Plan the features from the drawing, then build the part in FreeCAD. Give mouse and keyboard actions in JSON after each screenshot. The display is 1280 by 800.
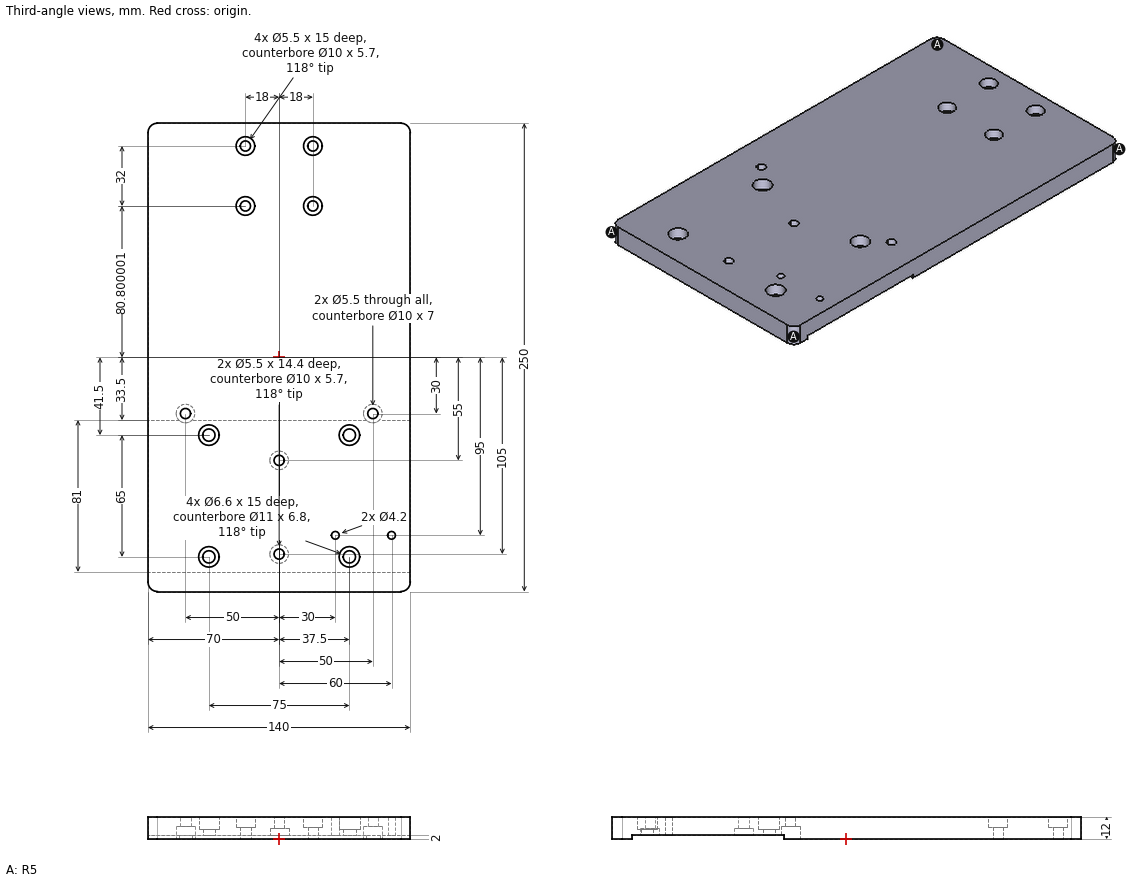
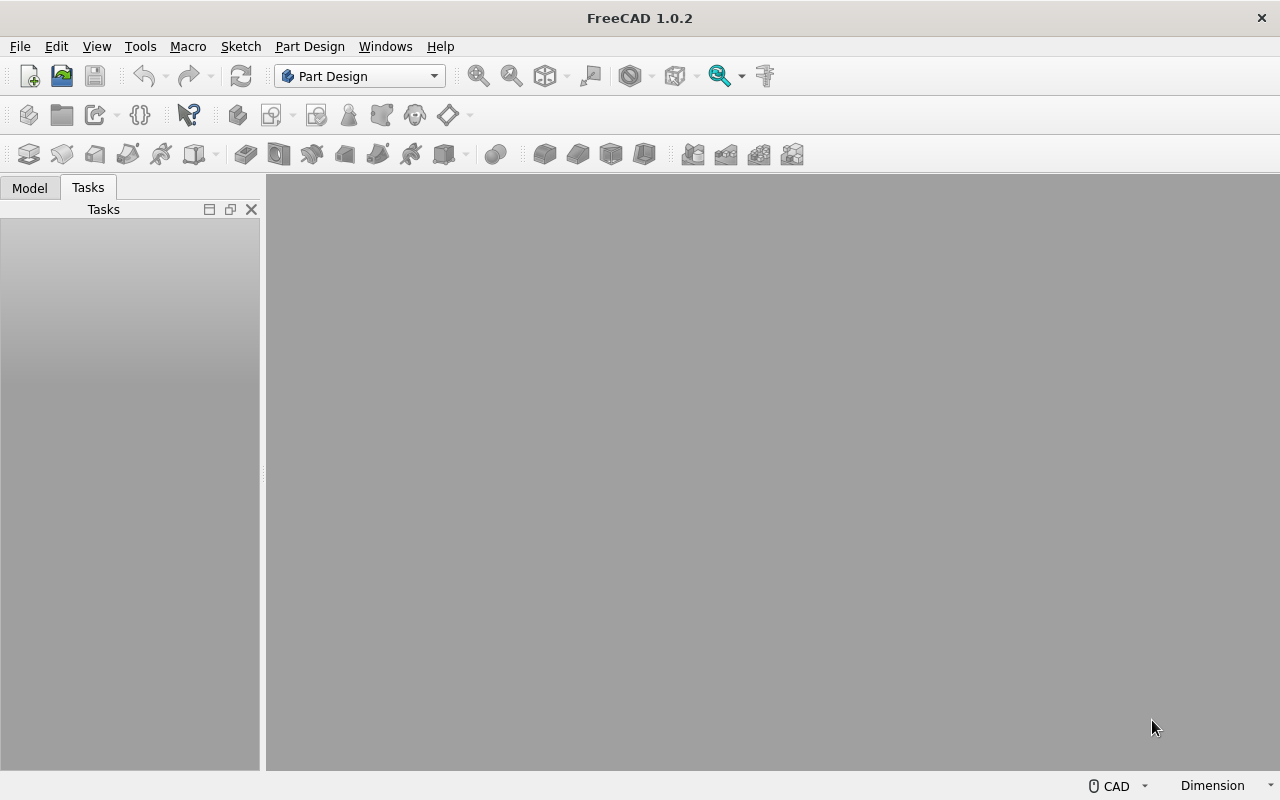
{"action": "left_click", "coordinate": [29, 76]}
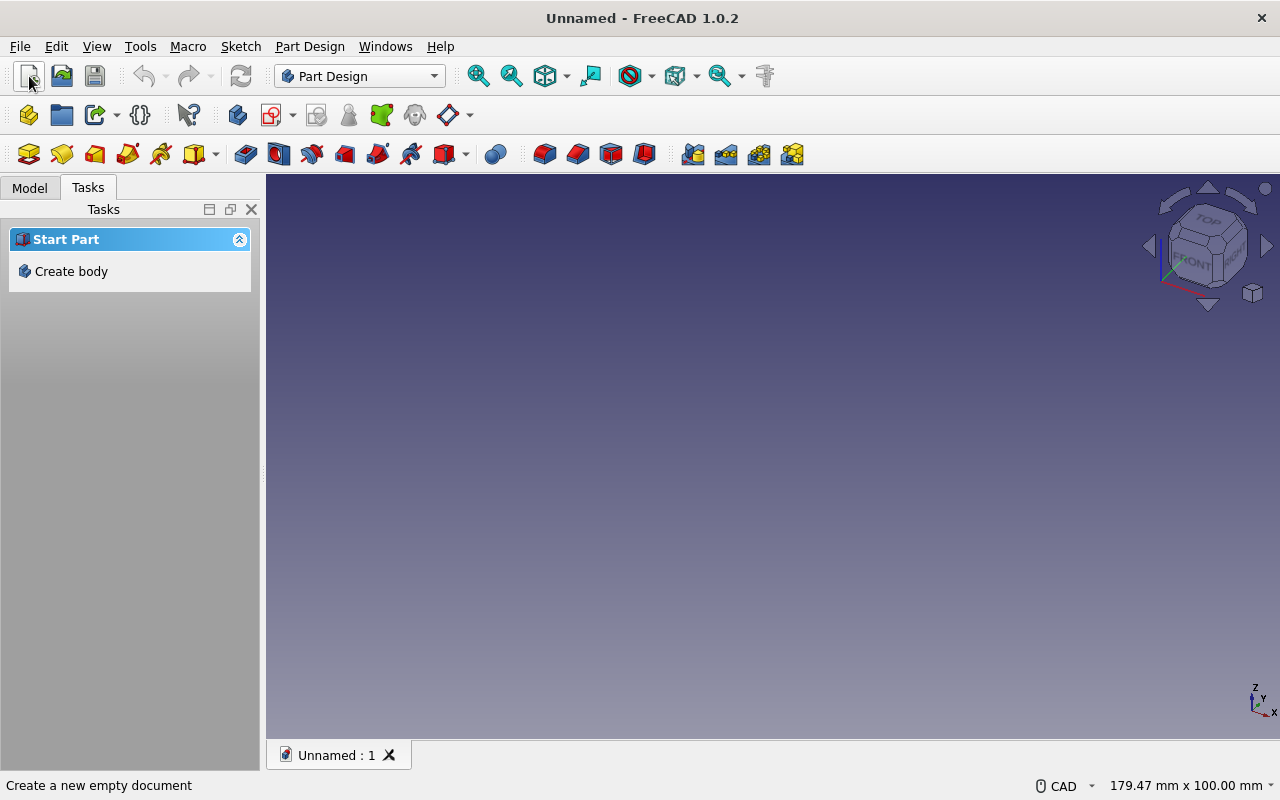
{"action": "left_click", "coordinate": [270, 116]}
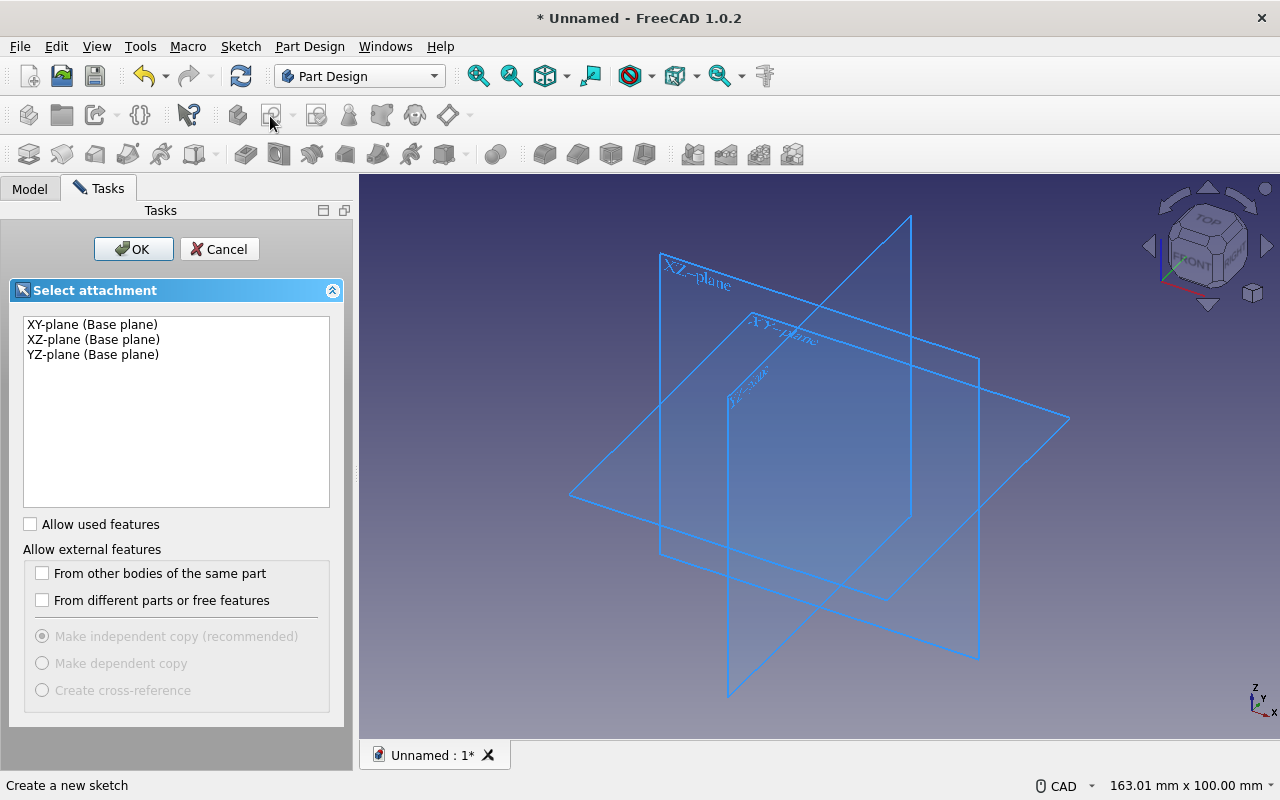
{"action": "left_click", "coordinate": [84, 324]}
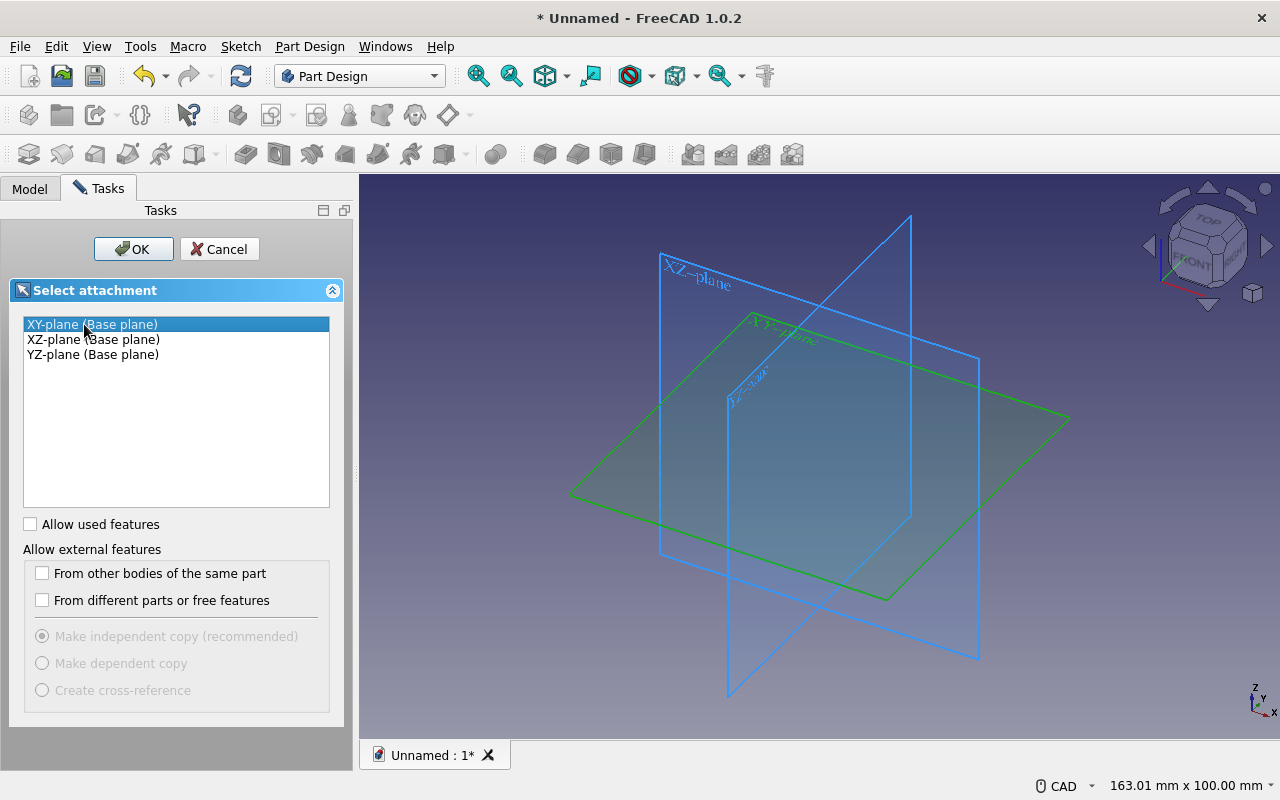
{"action": "left_click", "coordinate": [134, 249]}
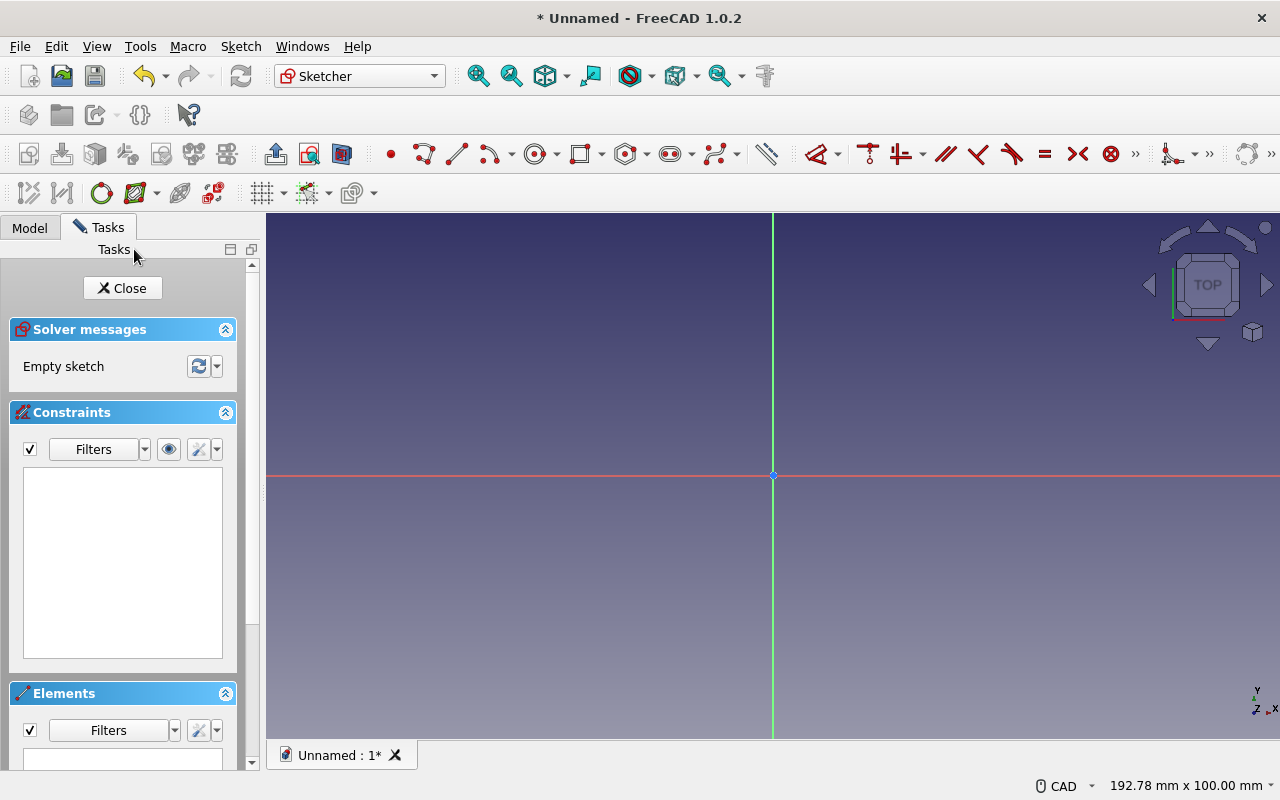
{"action": "scroll", "coordinate": [682, 476], "scroll_direction": "down", "scroll_amount": 7}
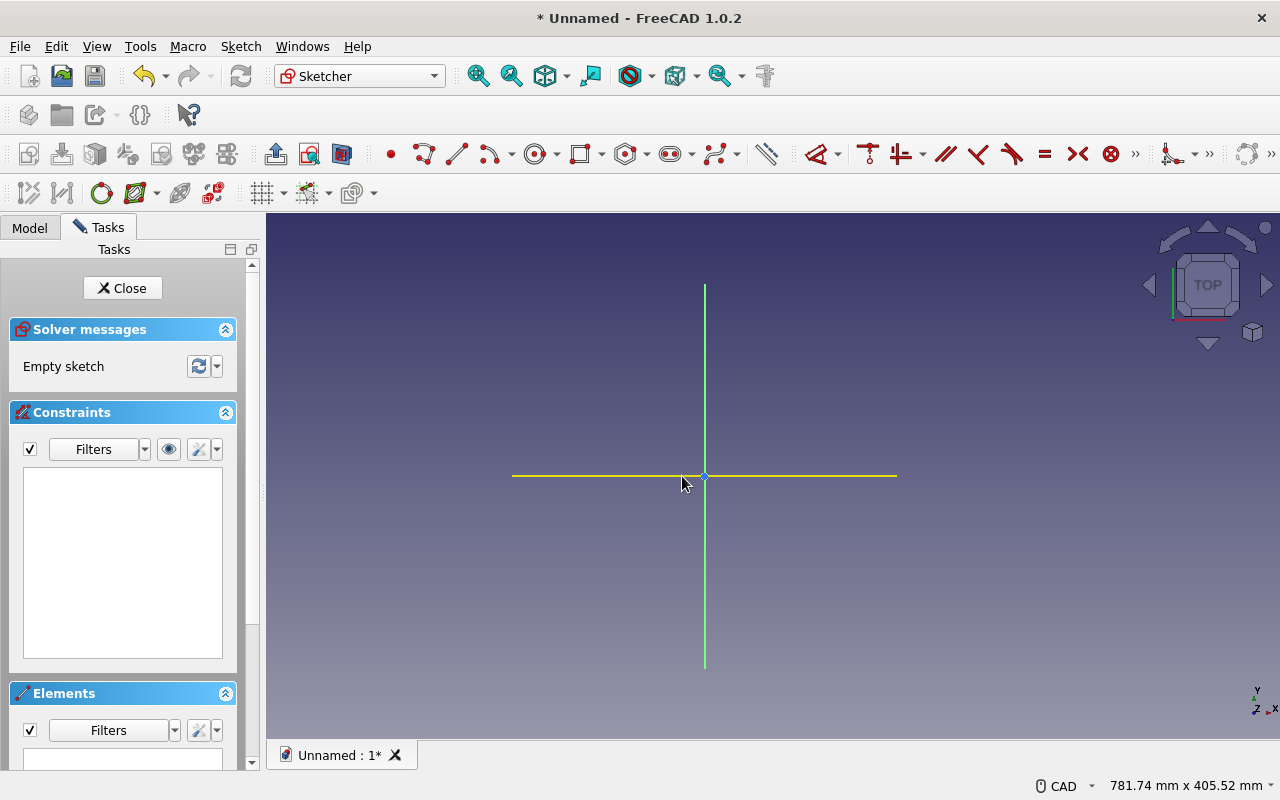
{"action": "left_click", "coordinate": [602, 154]}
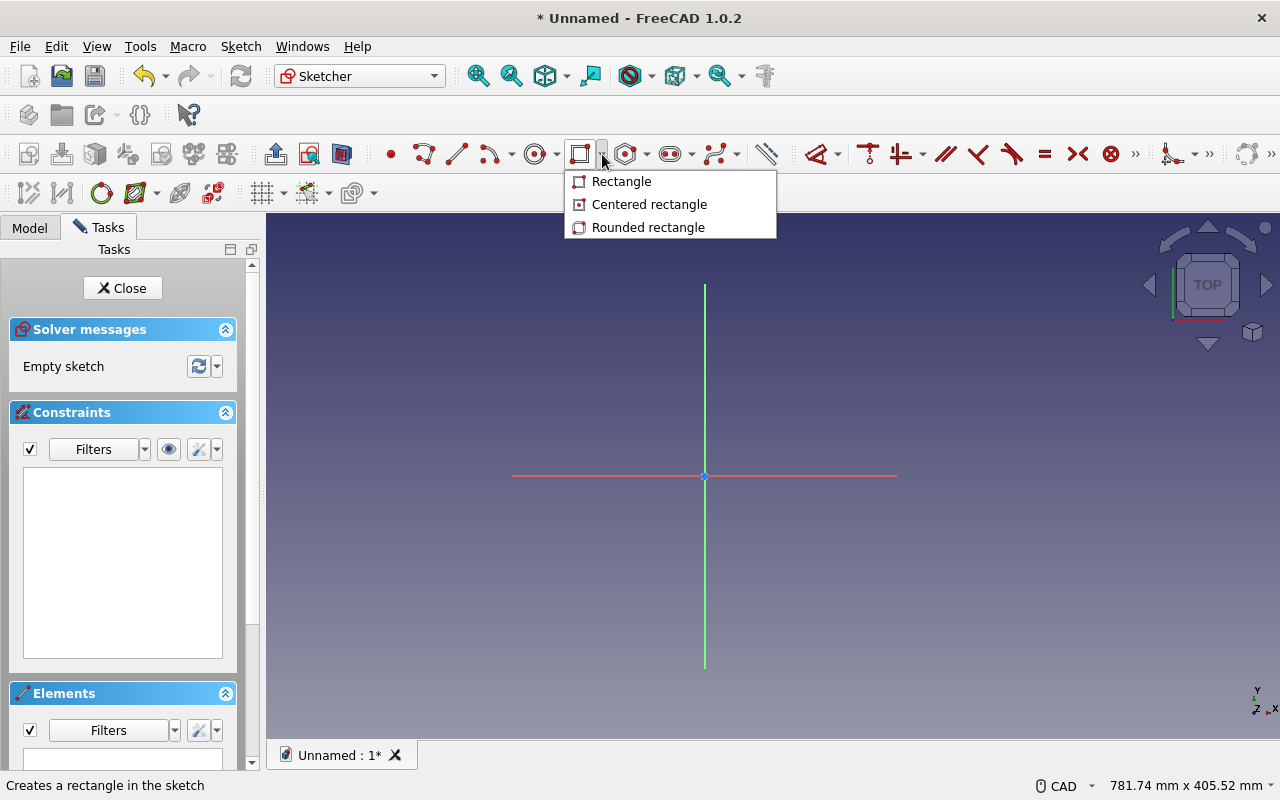
{"action": "left_click", "coordinate": [670, 204]}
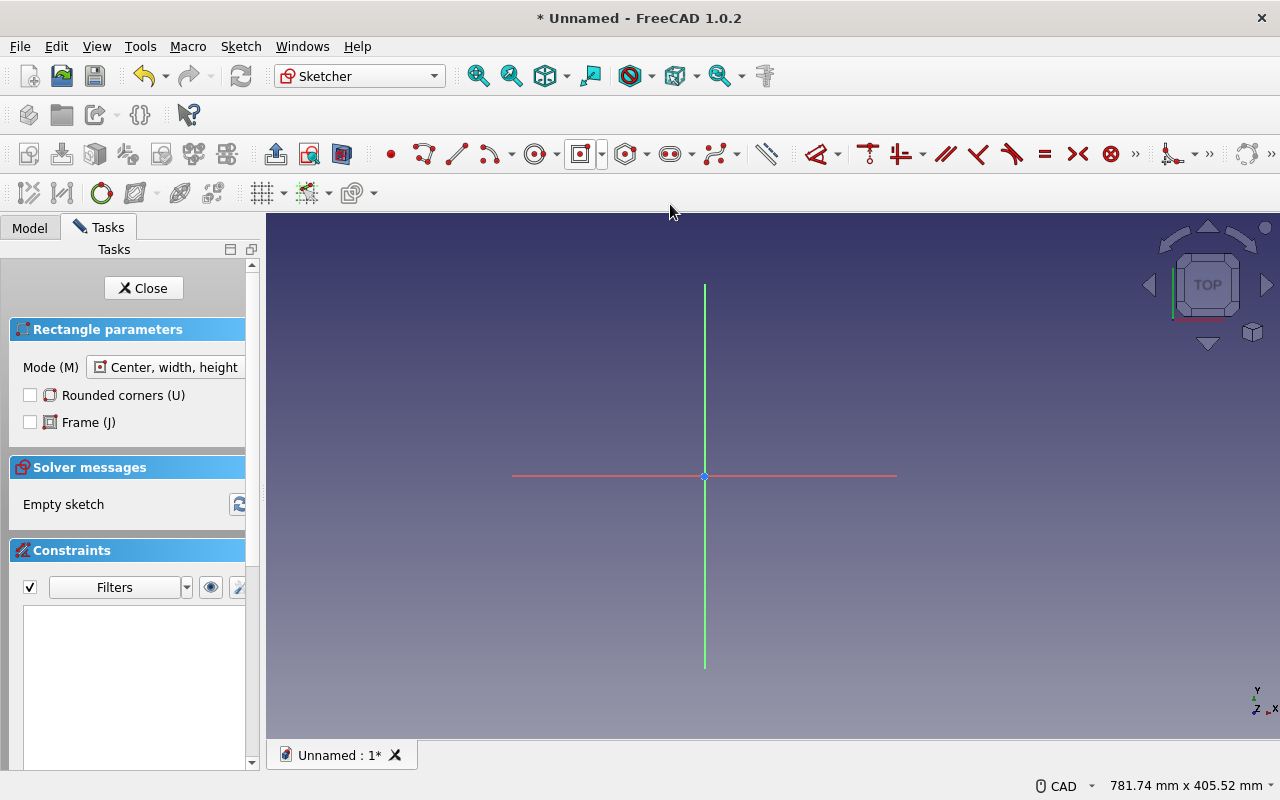
{"action": "left_click", "coordinate": [705, 476]}
{"action": "left_click", "coordinate": [796, 314]}
{"action": "key", "text": "Escape"}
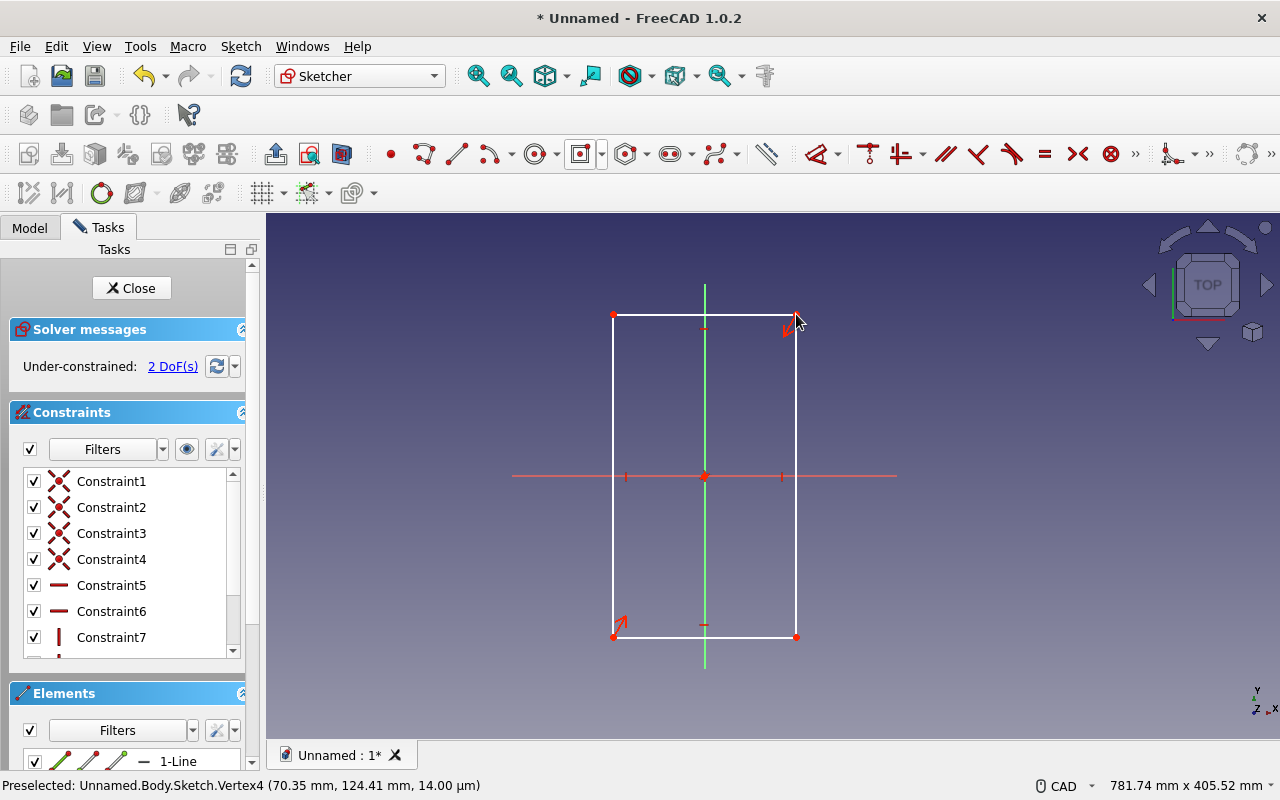
{"action": "left_click", "coordinate": [668, 638]}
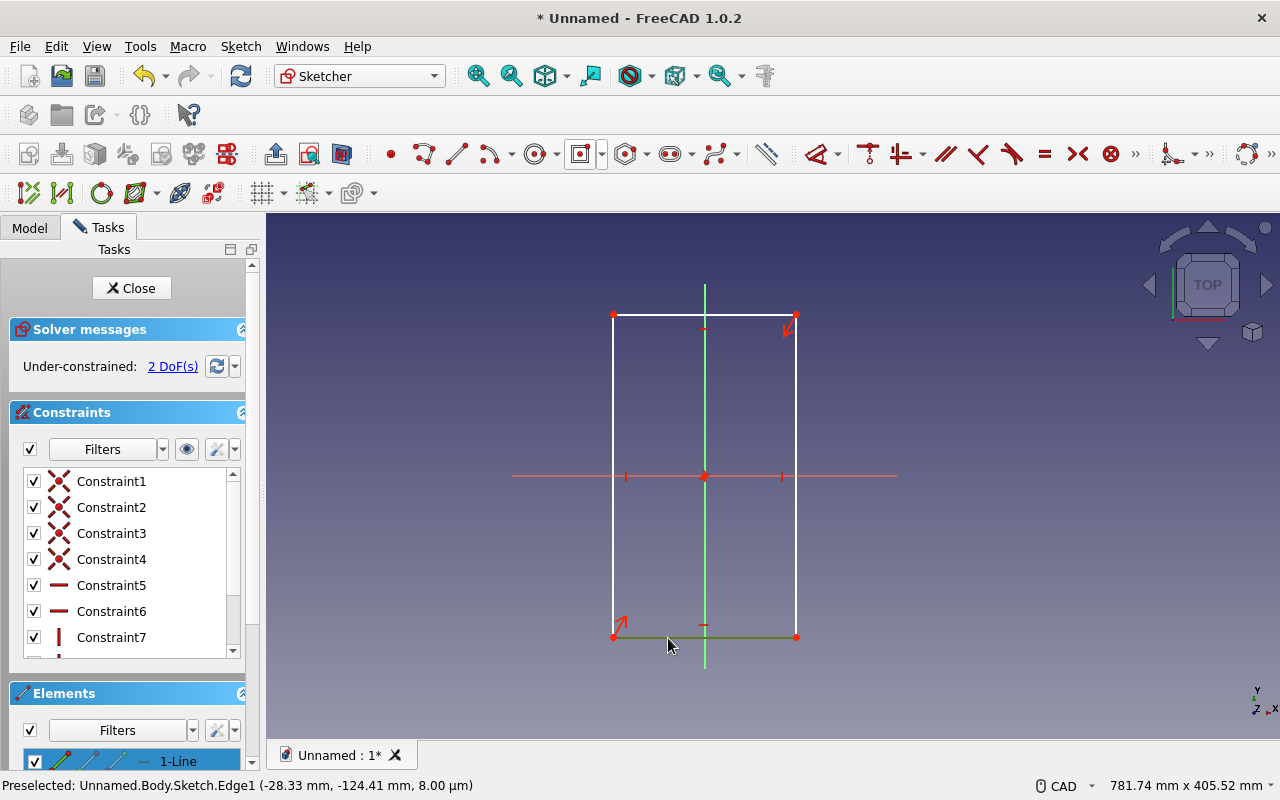
{"action": "key", "text": "l"}